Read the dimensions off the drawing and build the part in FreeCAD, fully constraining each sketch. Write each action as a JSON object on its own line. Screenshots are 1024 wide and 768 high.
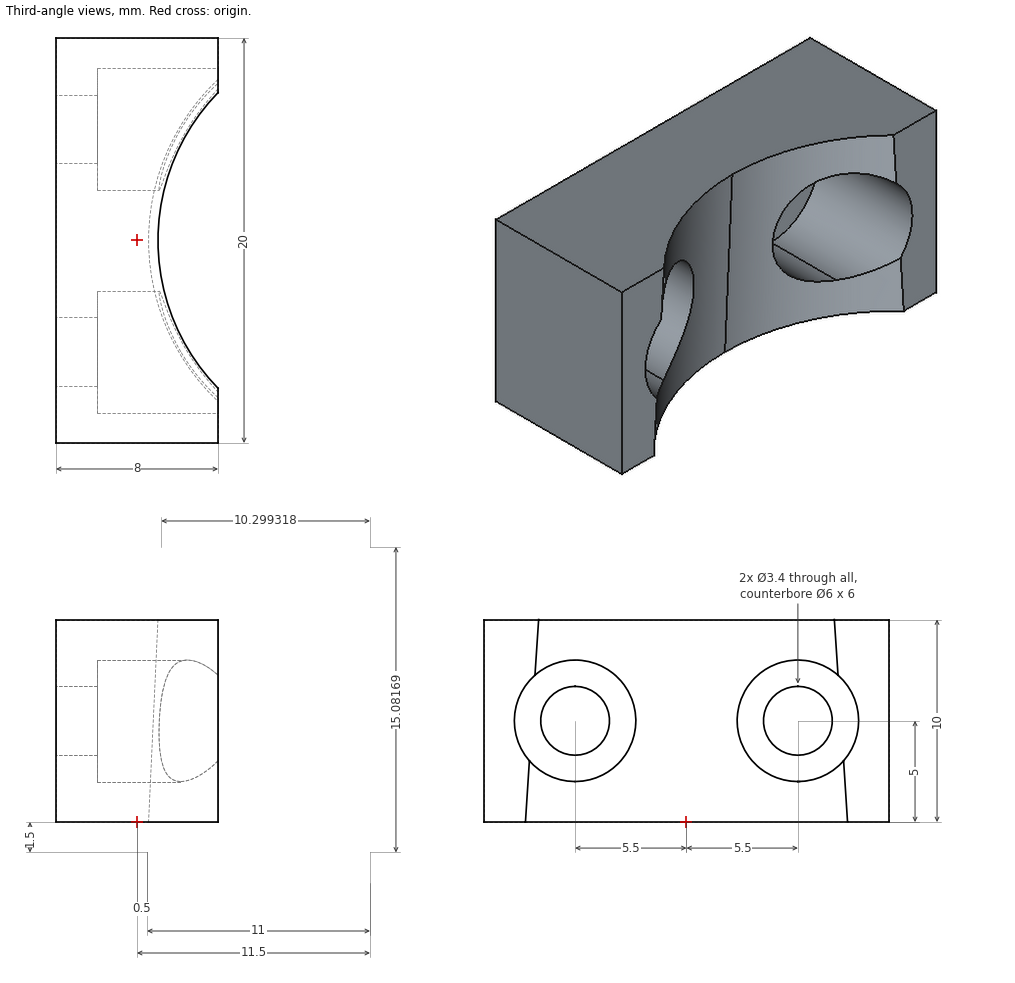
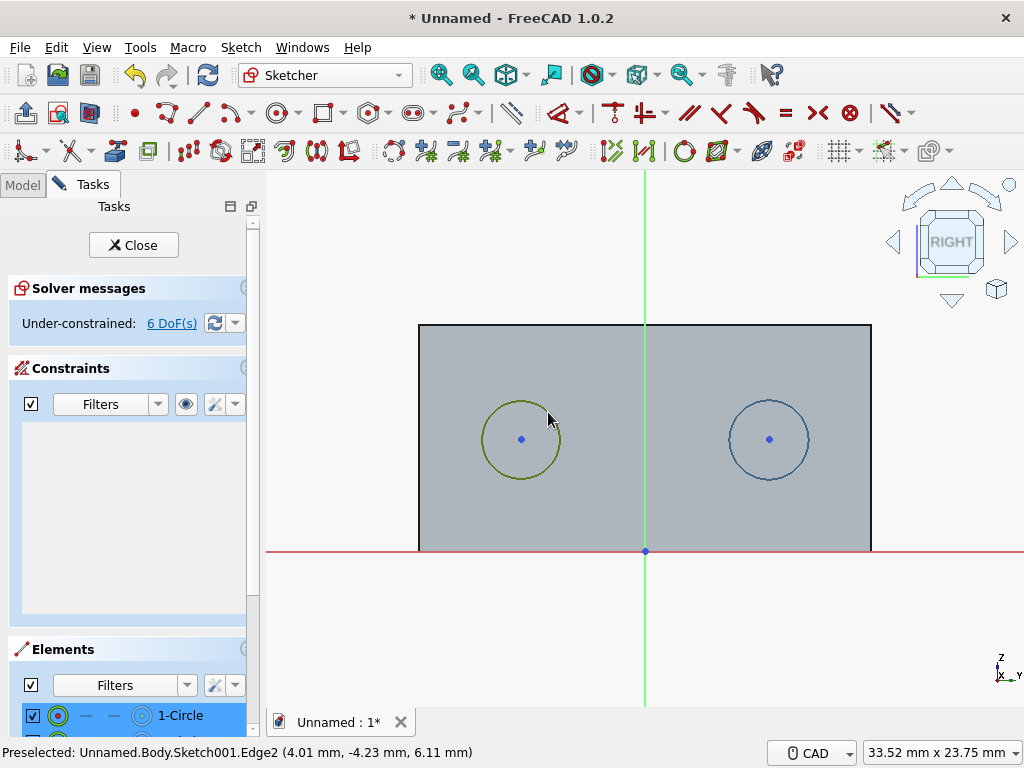
{"action": "key", "text": "e"}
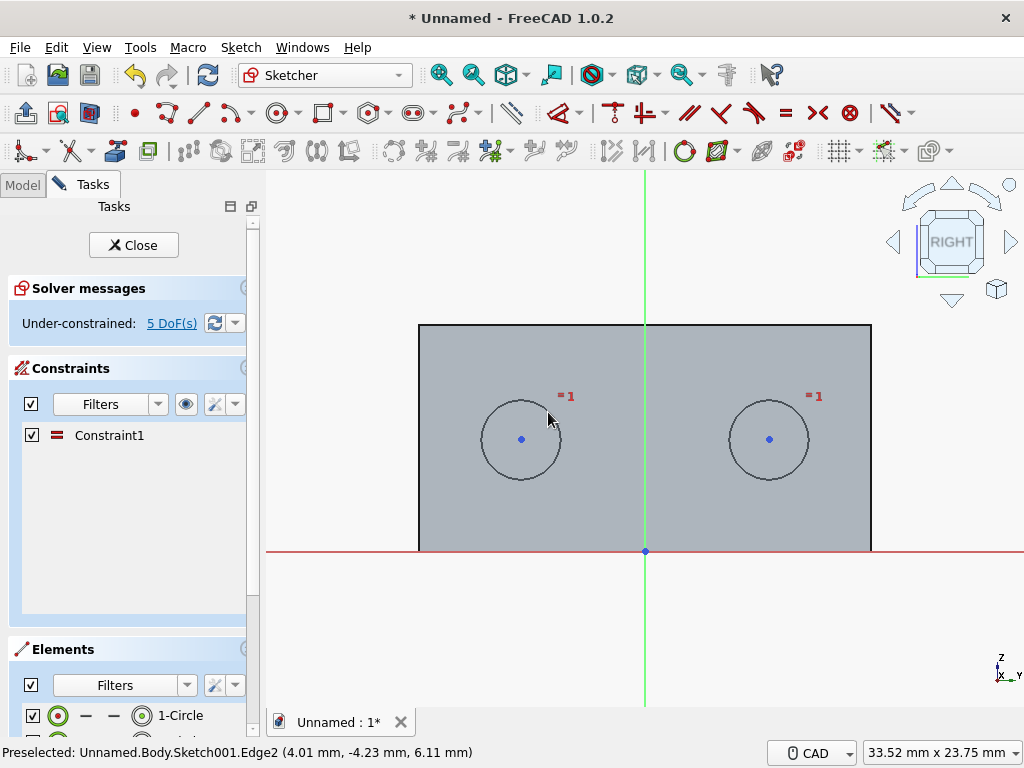
{"action": "key", "text": "d"}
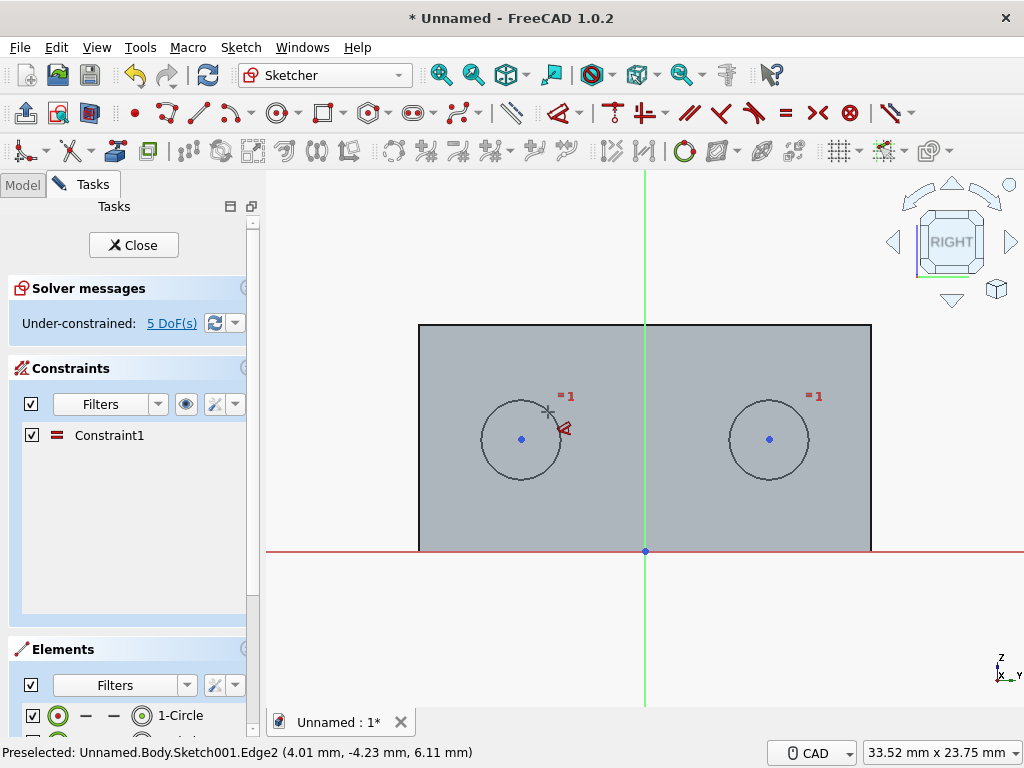
{"action": "left_click", "coordinate": [797, 412]}
{"action": "left_click", "coordinate": [820, 389]}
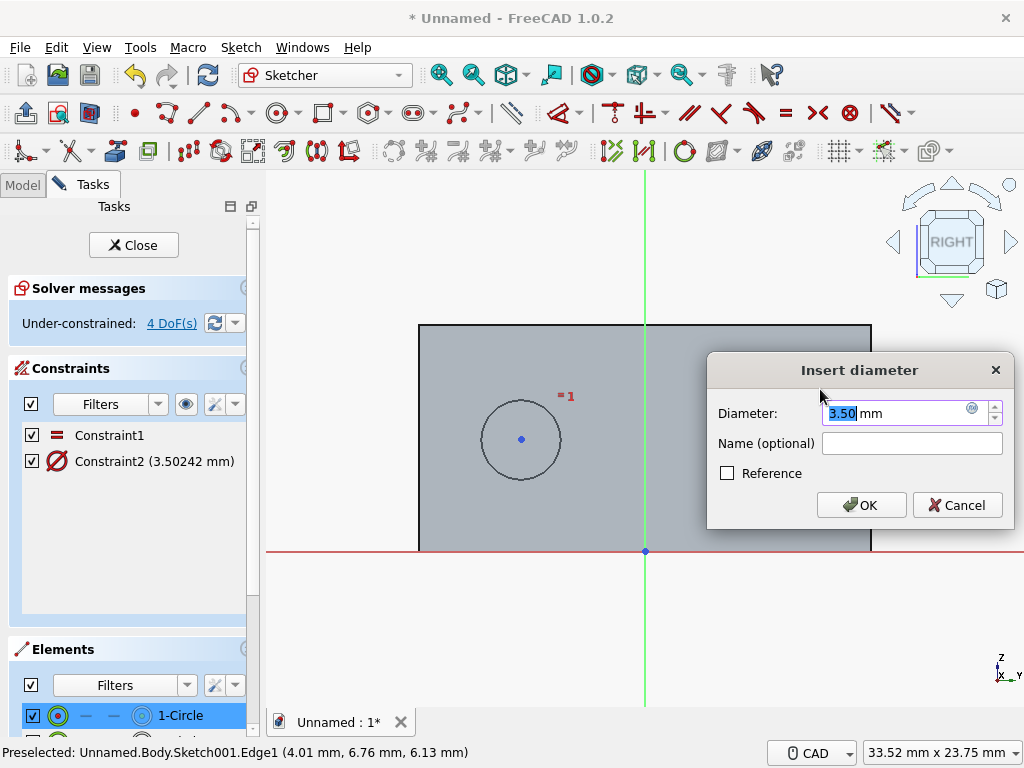
{"action": "type", "text": "3.4"}
{"action": "key", "text": "Return"}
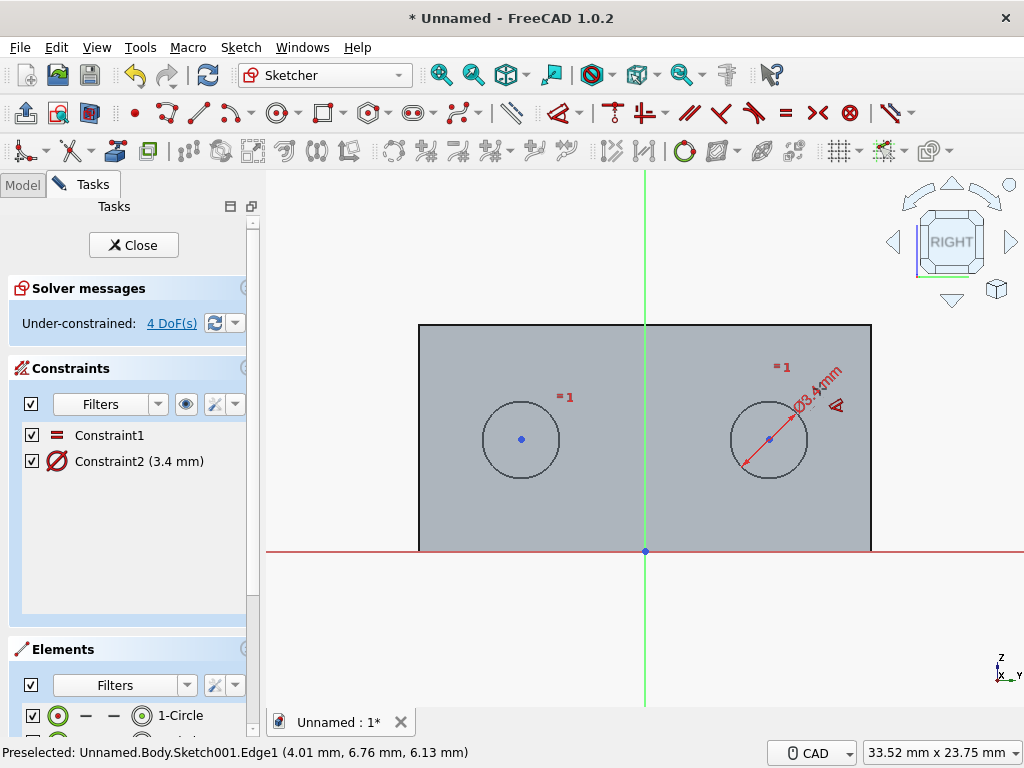
{"action": "left_click", "coordinate": [769, 440]}
{"action": "left_click", "coordinate": [803, 496]}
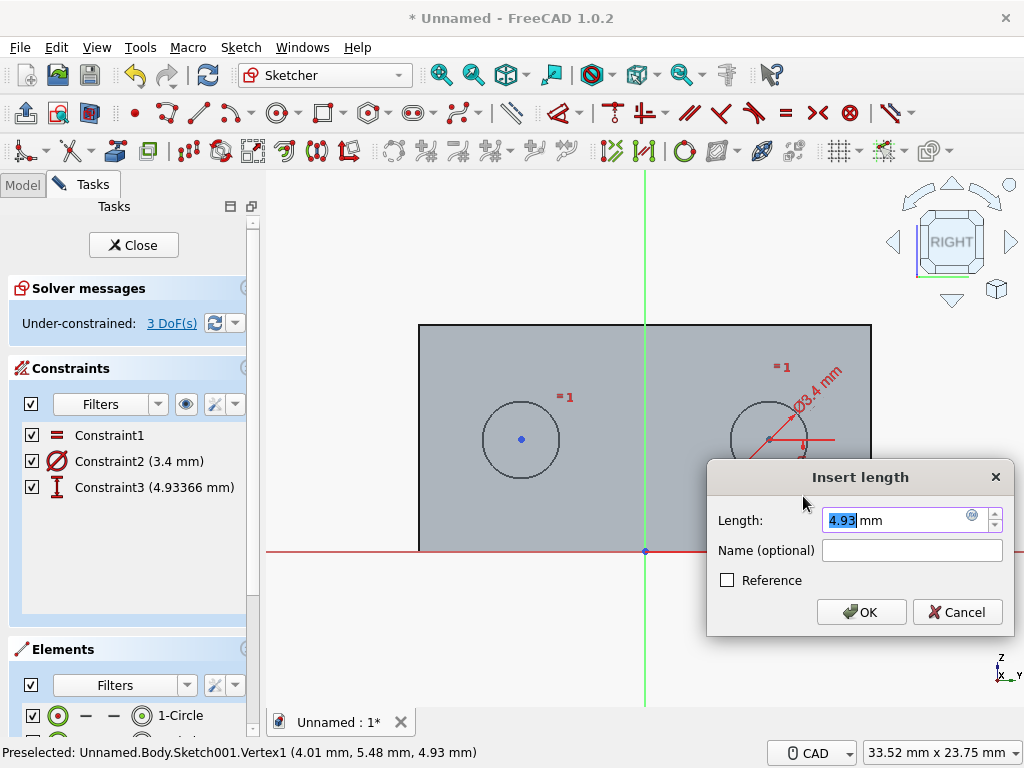
{"action": "type", "text": "5"}
{"action": "key", "text": "Return"}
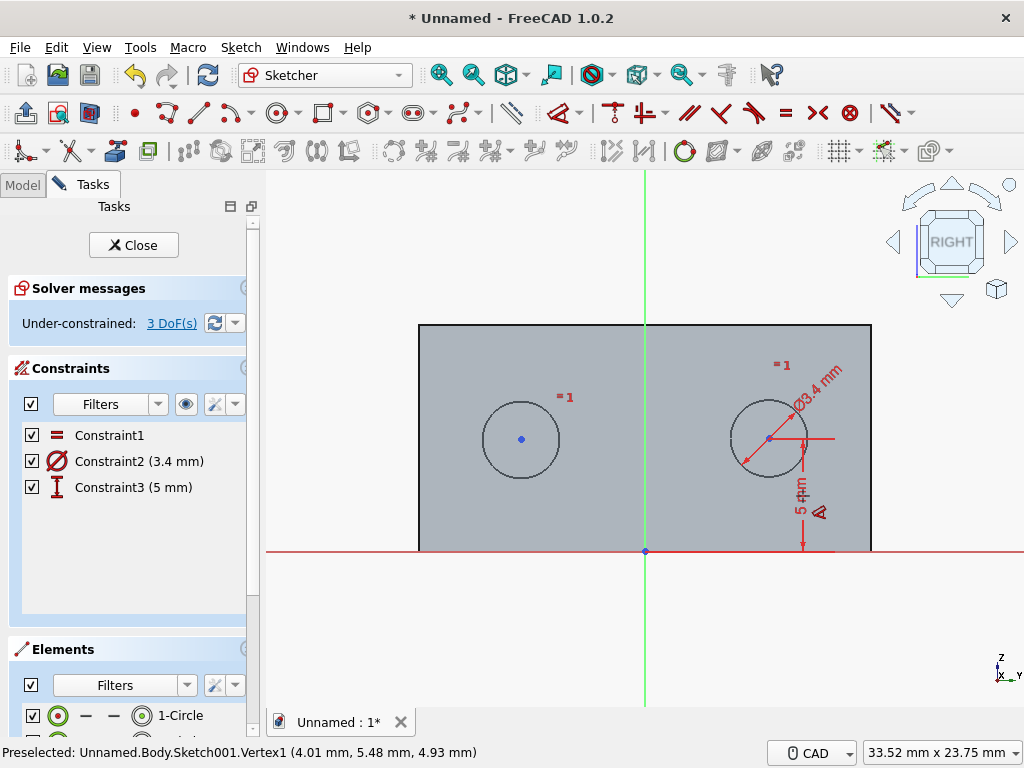
{"action": "left_click", "coordinate": [521, 440]}
{"action": "left_click", "coordinate": [487, 496]}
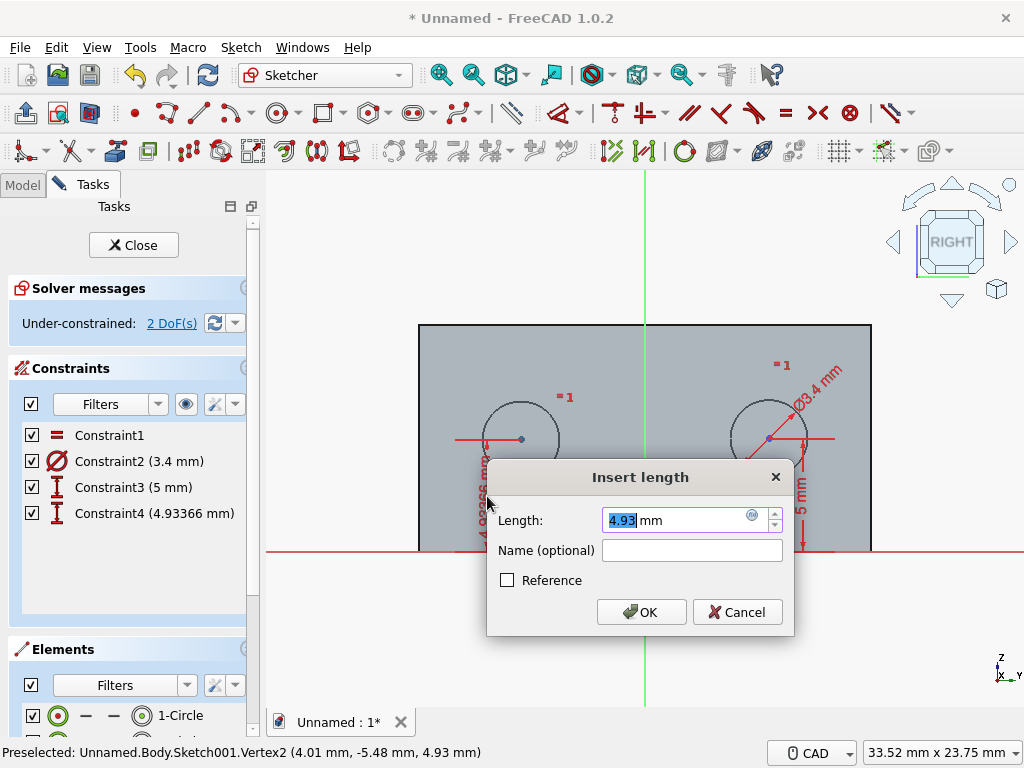
{"action": "type", "text": "5"}
{"action": "key", "text": "Return"}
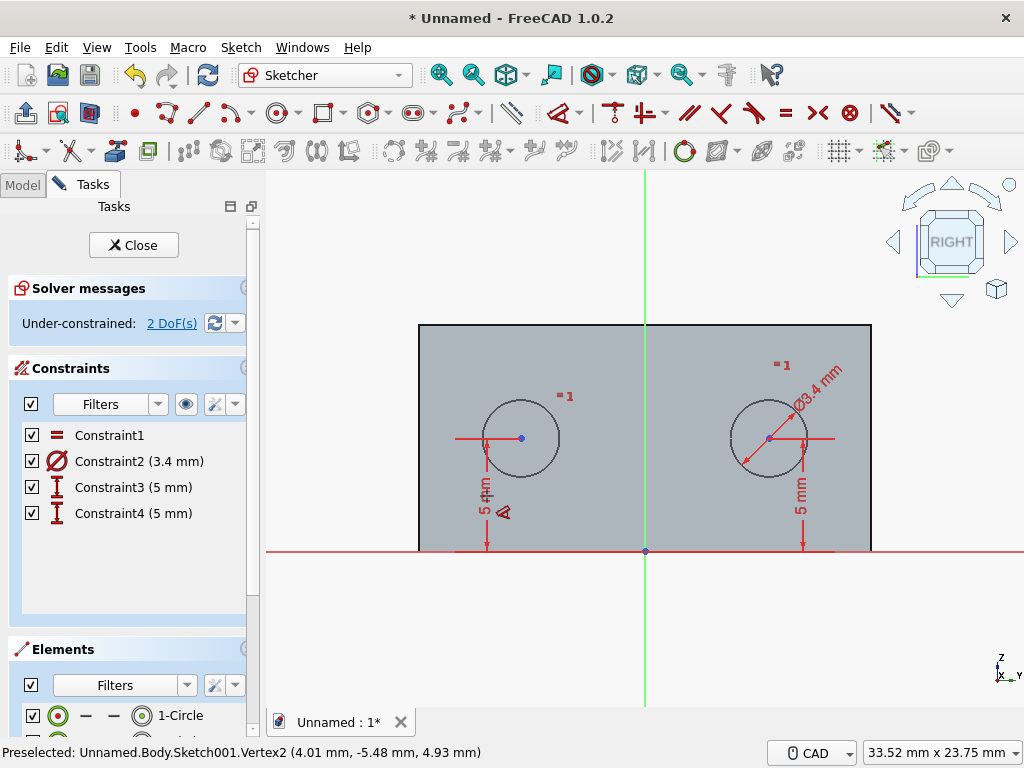
{"action": "left_click", "coordinate": [769, 439]}
{"action": "left_click", "coordinate": [707, 586]}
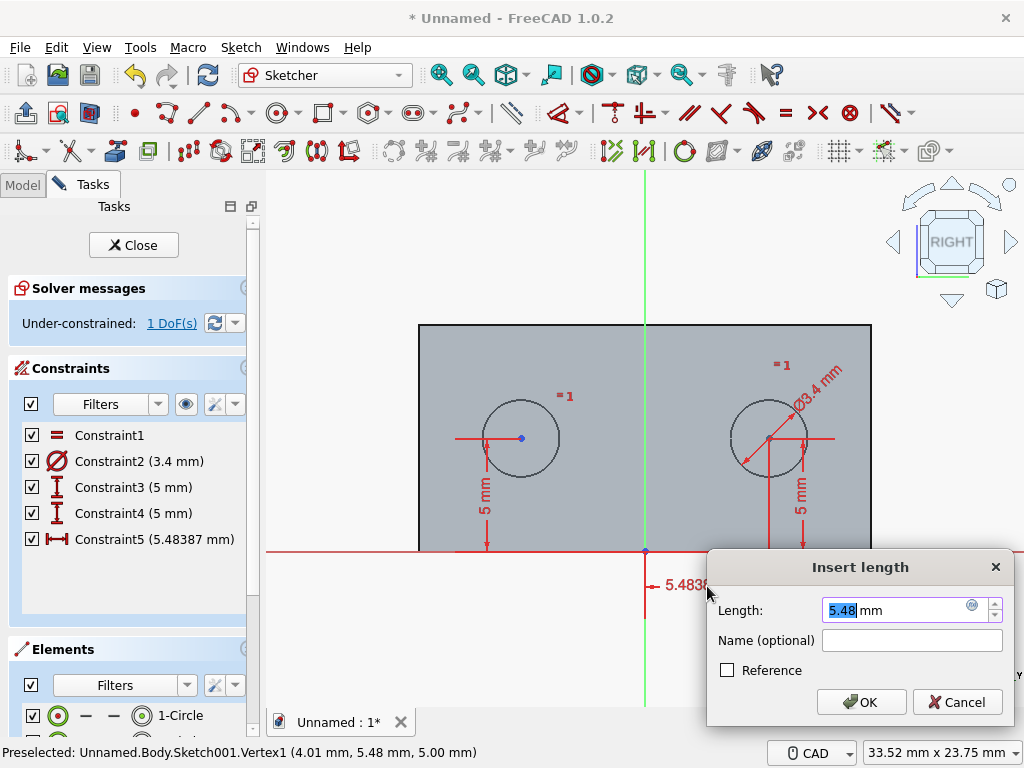
{"action": "type", "text": "5.5"}
{"action": "key", "text": "Return"}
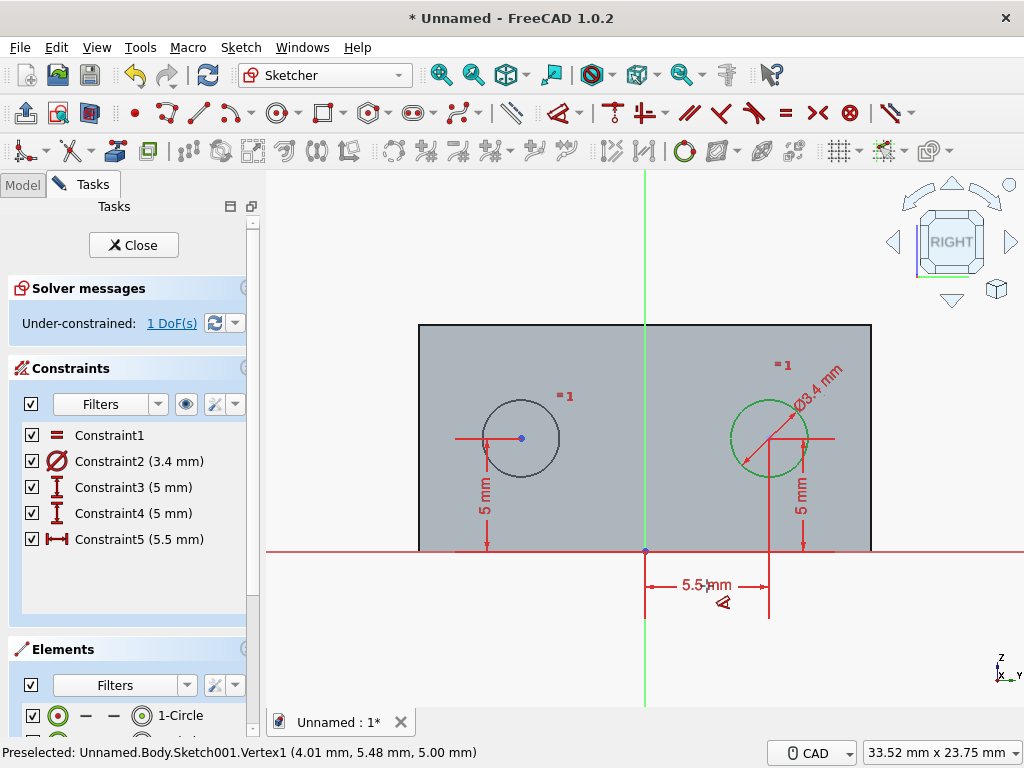
{"action": "left_click", "coordinate": [521, 439]}
{"action": "left_click", "coordinate": [583, 586]}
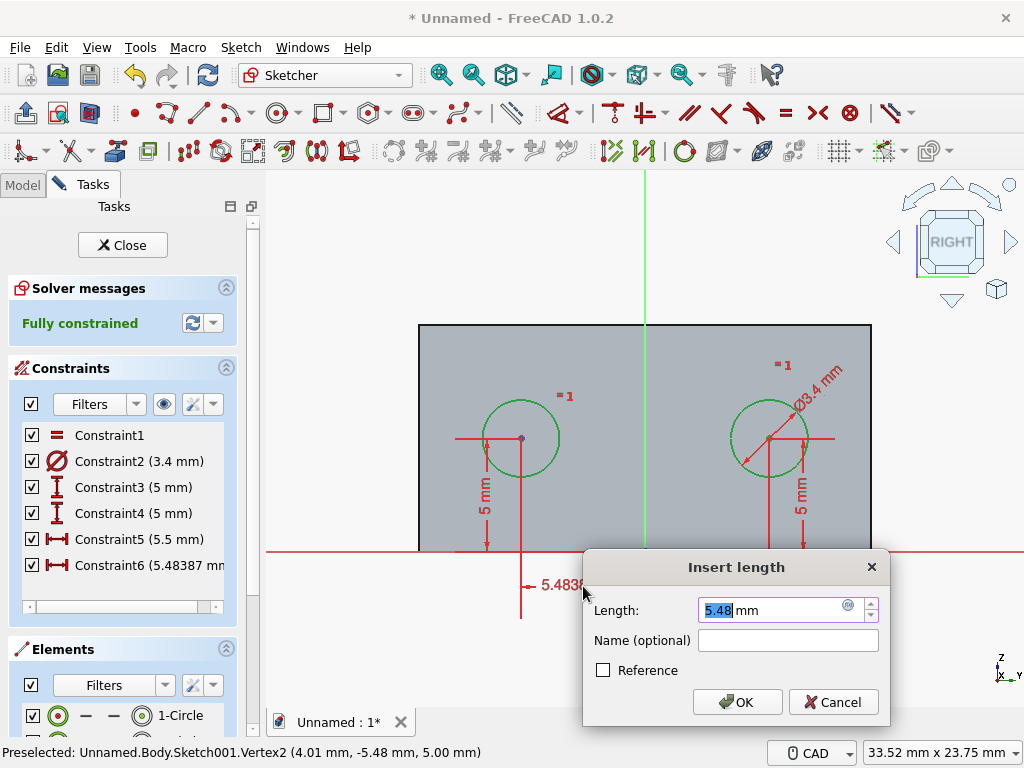
{"action": "type", "text": "5.5"}
{"action": "key", "text": "Return"}
{"action": "key", "text": "Escape"}